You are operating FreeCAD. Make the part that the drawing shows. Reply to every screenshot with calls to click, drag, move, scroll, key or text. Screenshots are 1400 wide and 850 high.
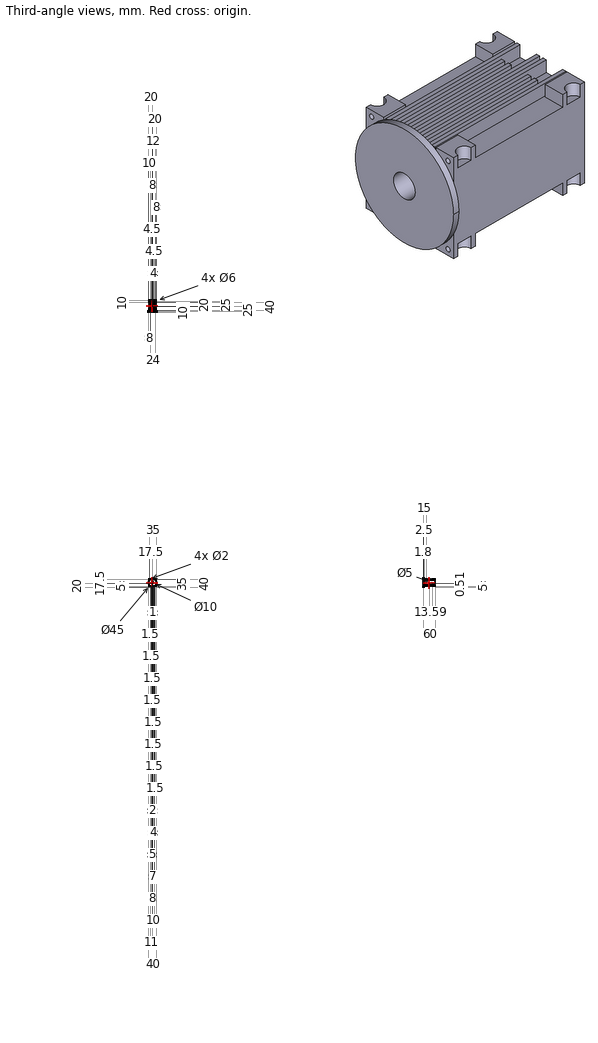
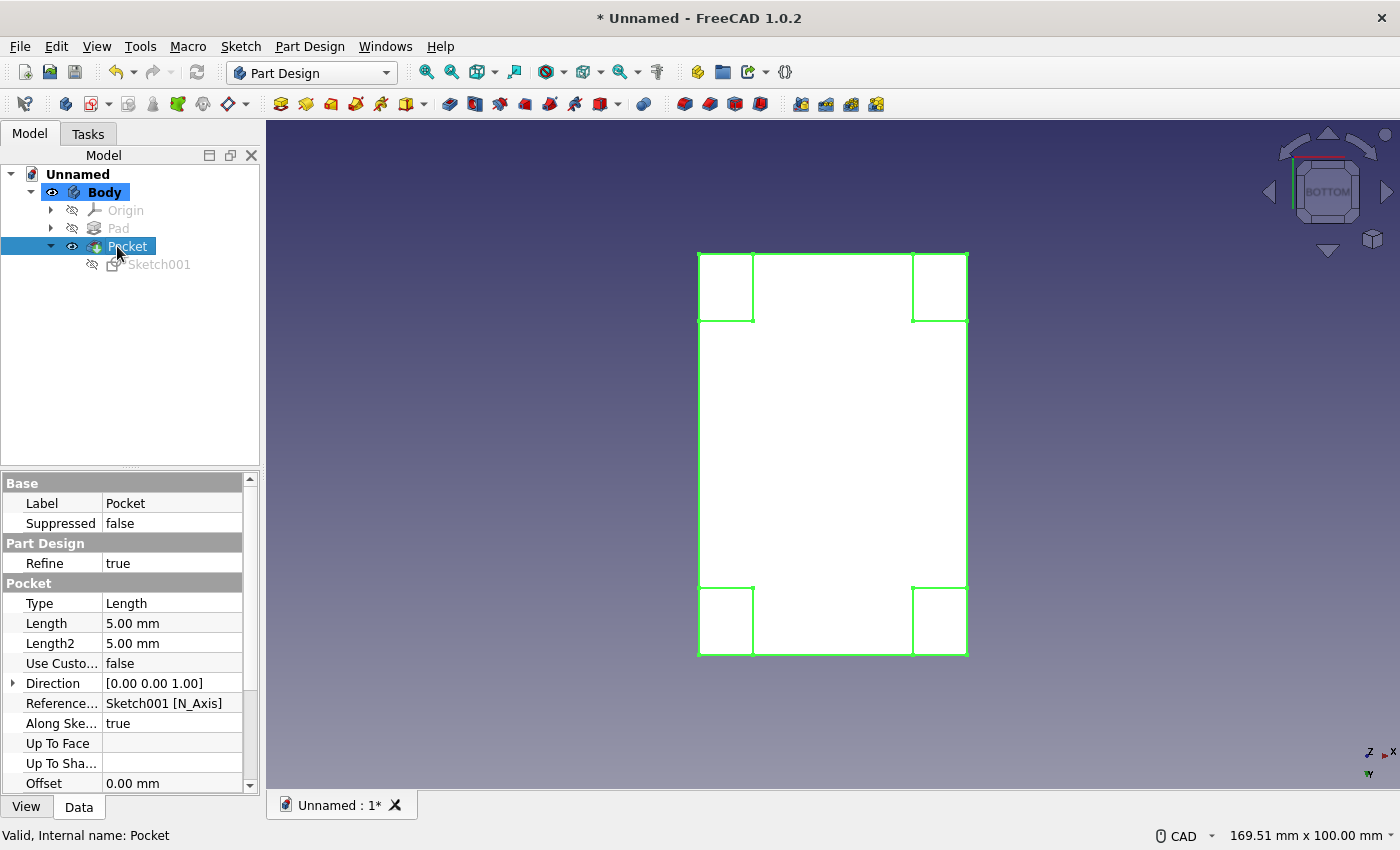
click(801, 104)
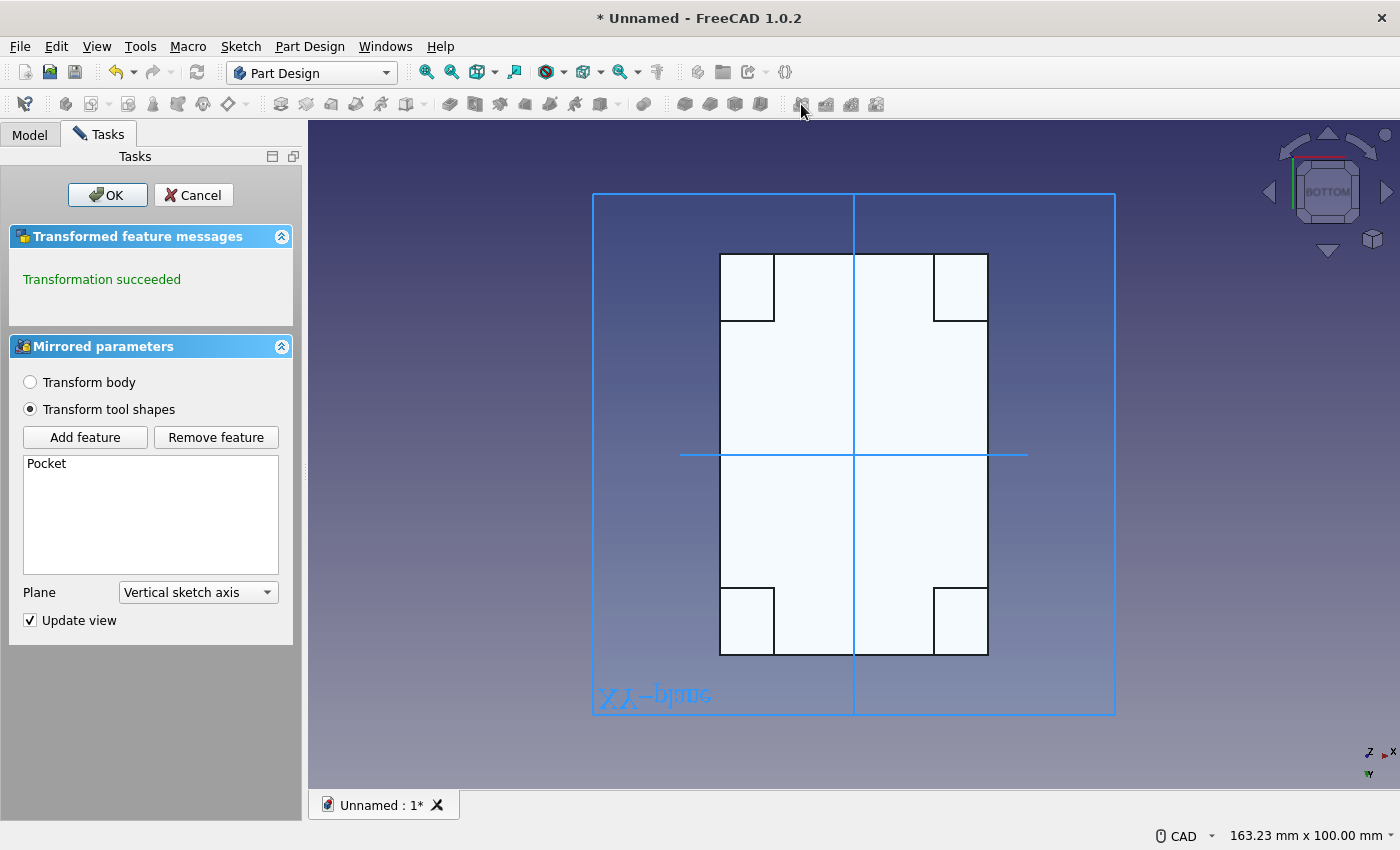
click(199, 592)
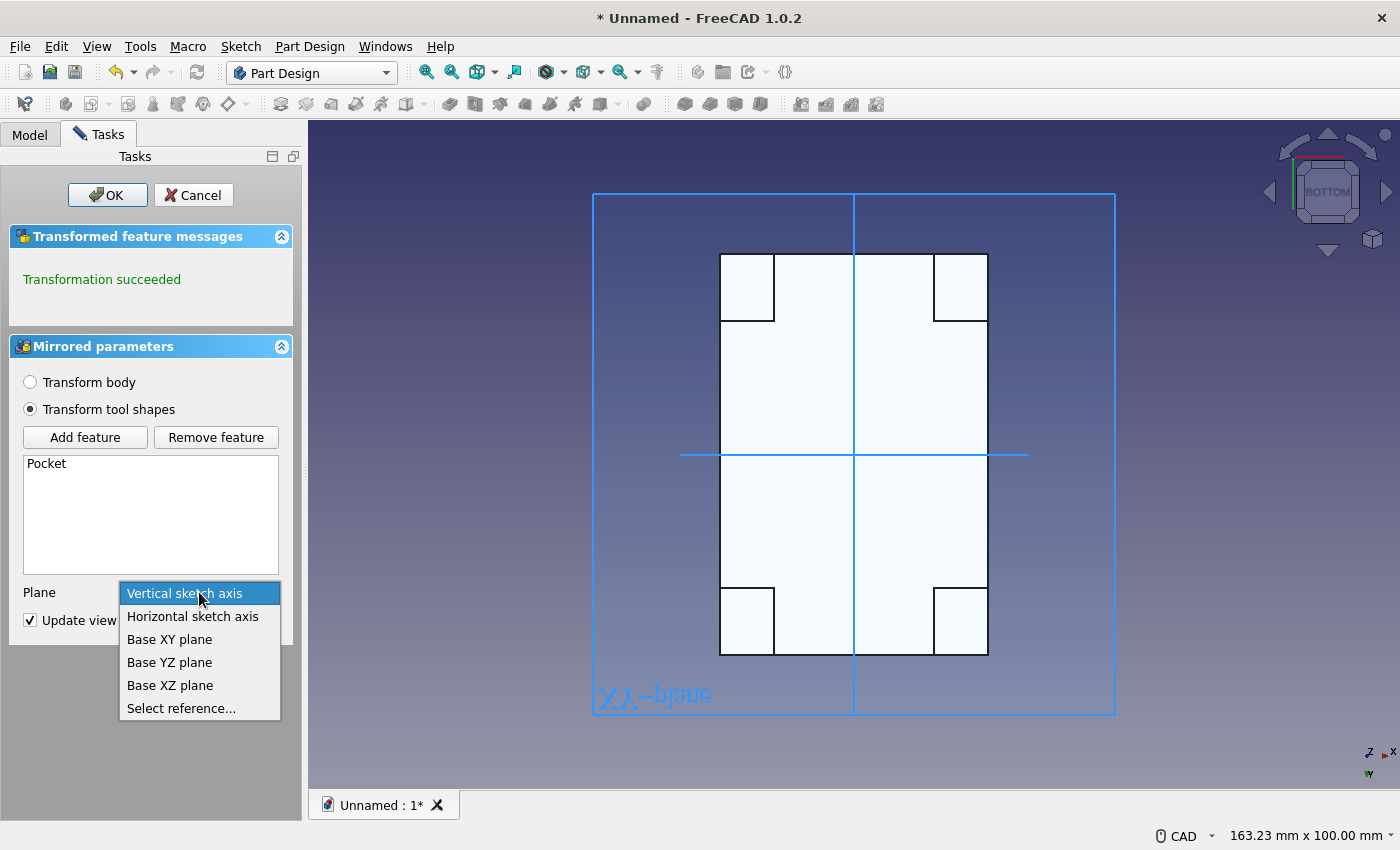
click(198, 640)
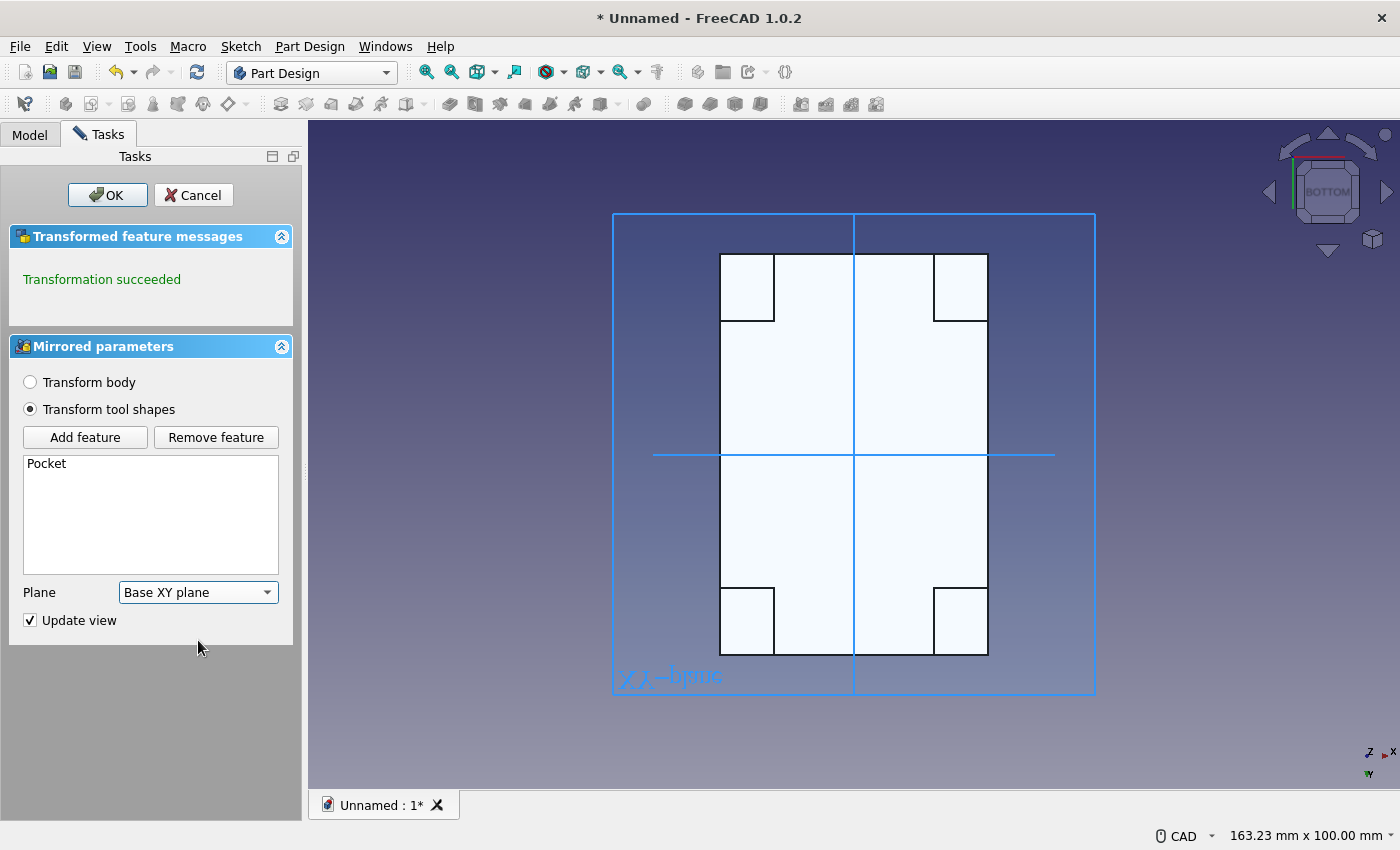
click(108, 195)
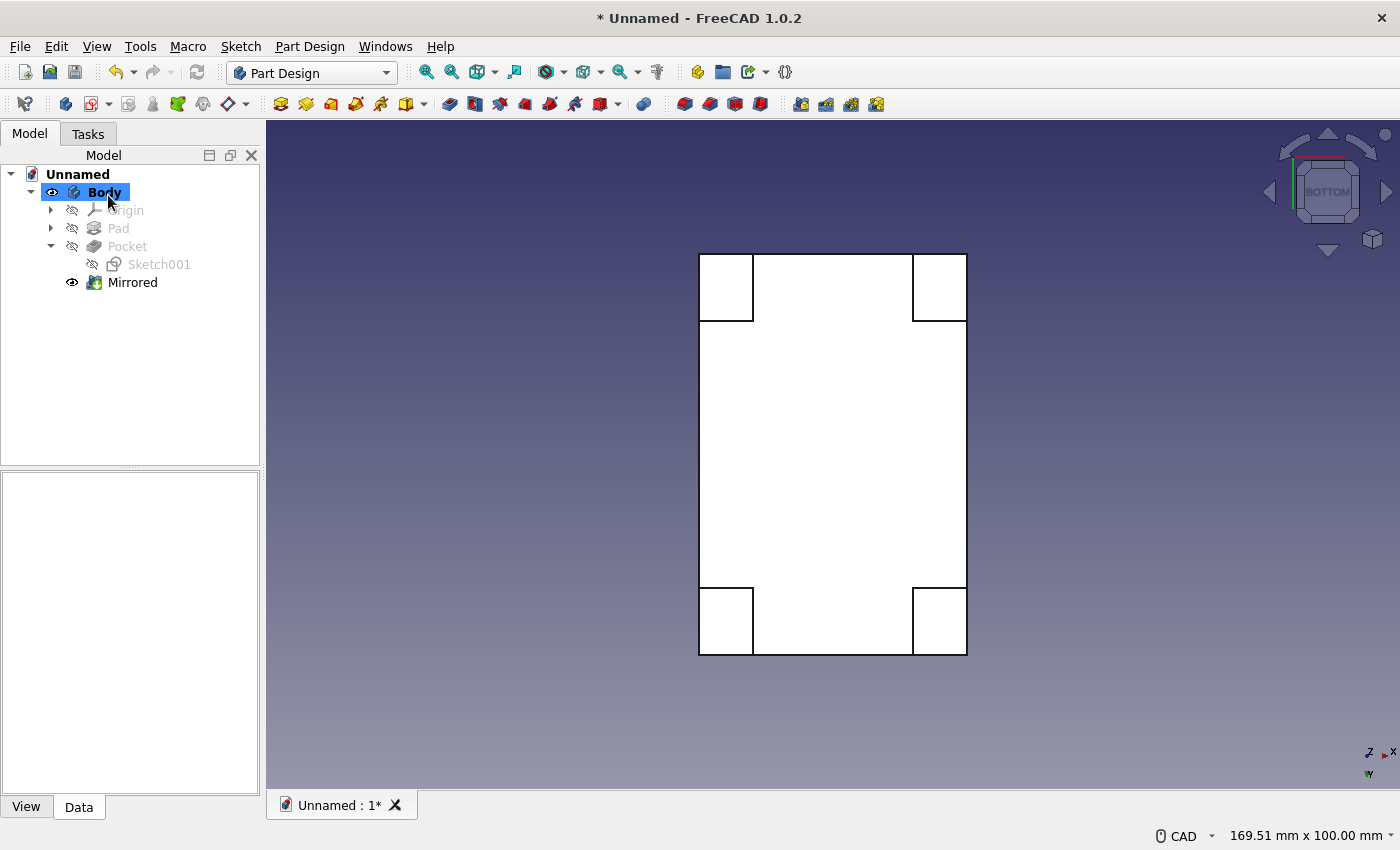
key(4)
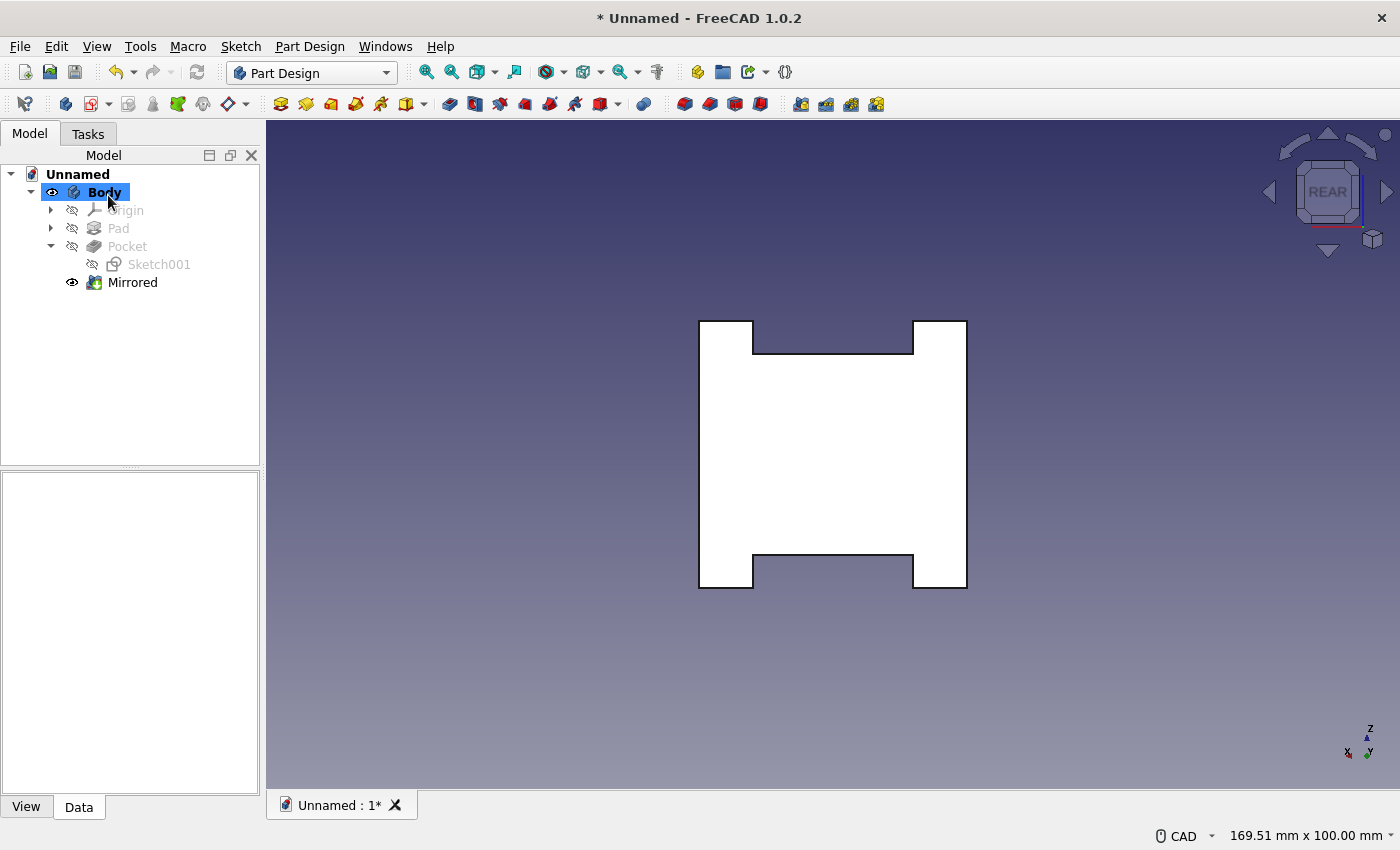
click(427, 72)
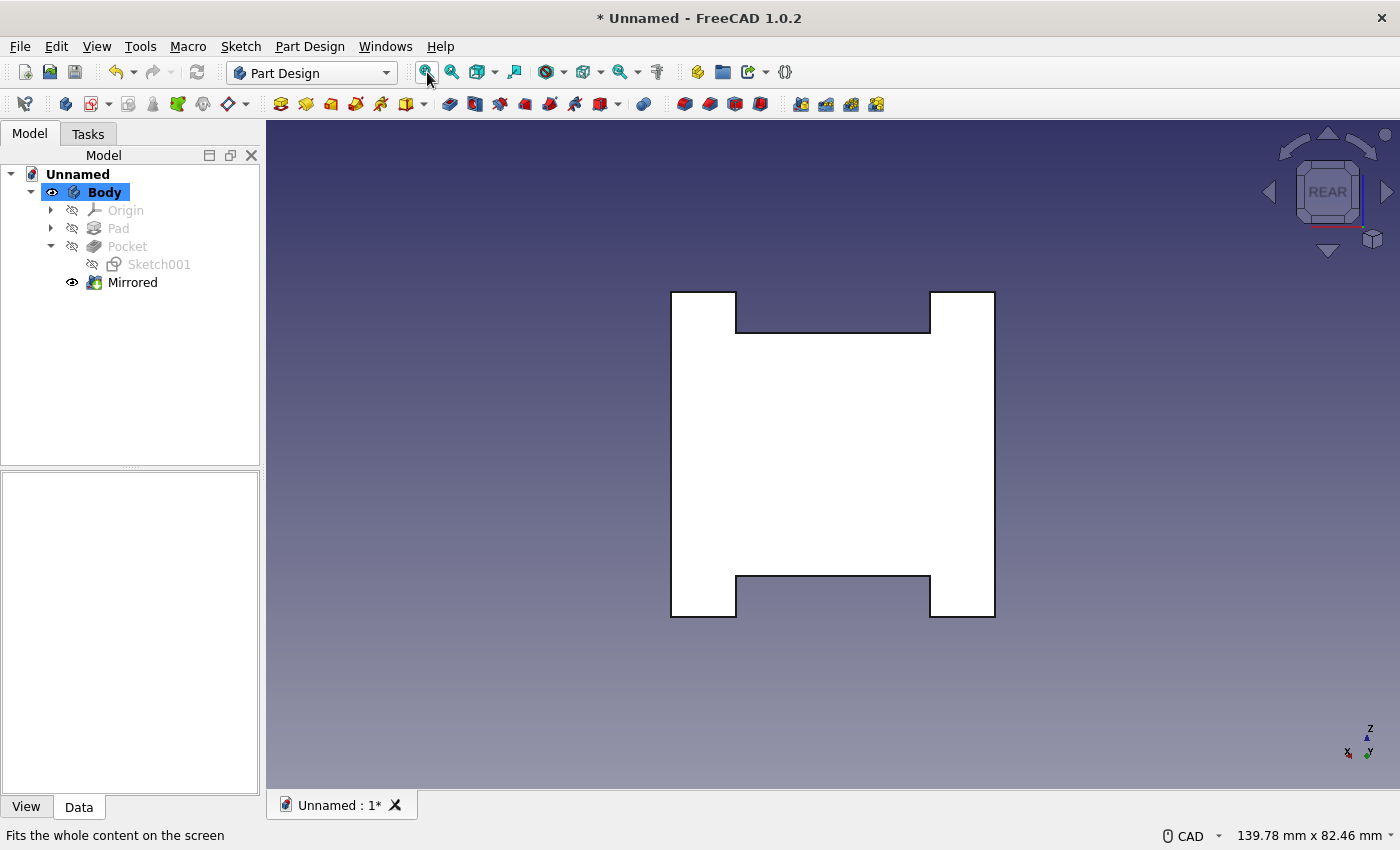
click(833, 454)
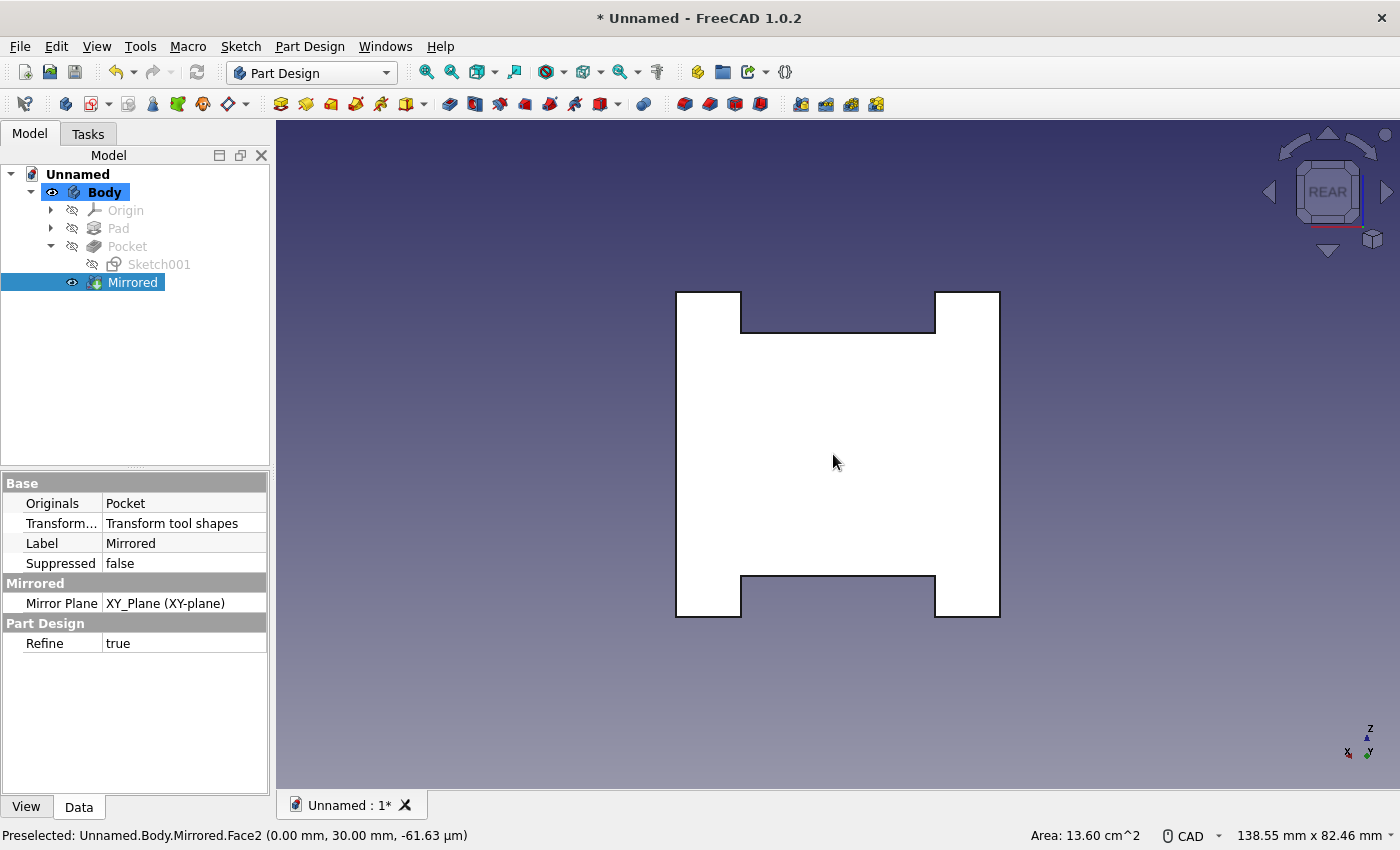
click(90, 104)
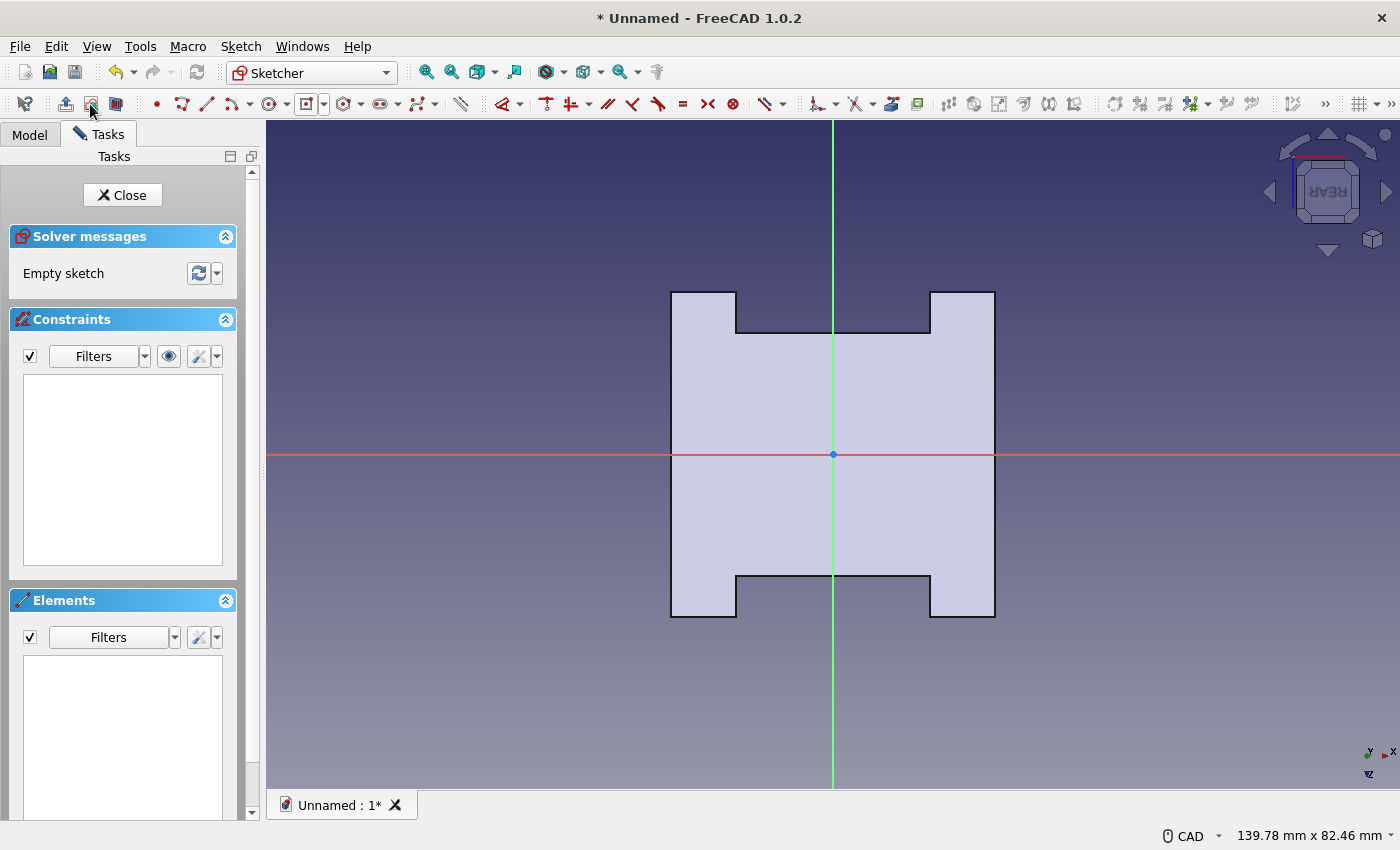
scroll(876, 326, up, 5)